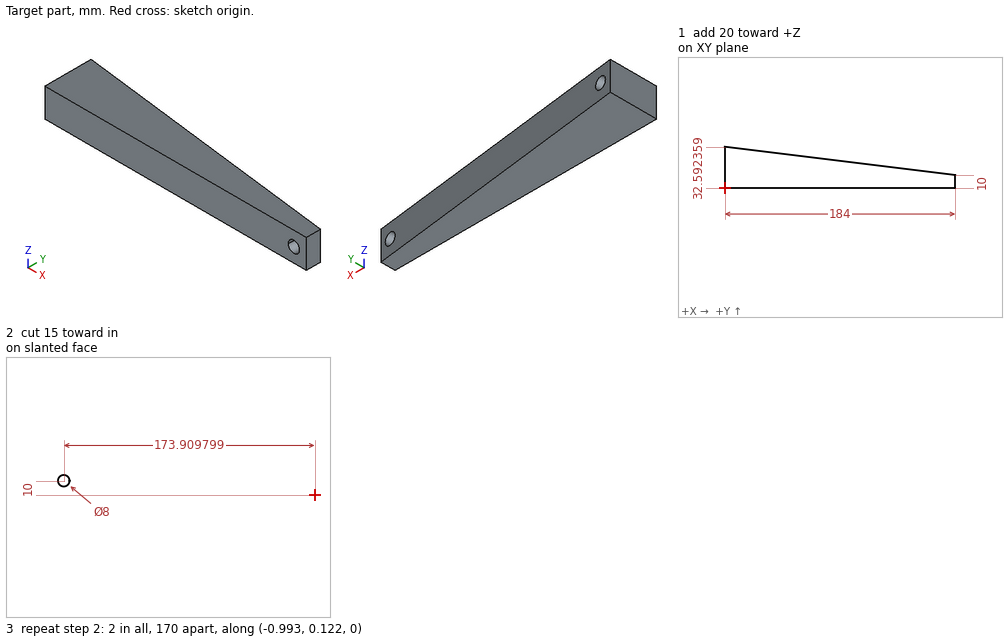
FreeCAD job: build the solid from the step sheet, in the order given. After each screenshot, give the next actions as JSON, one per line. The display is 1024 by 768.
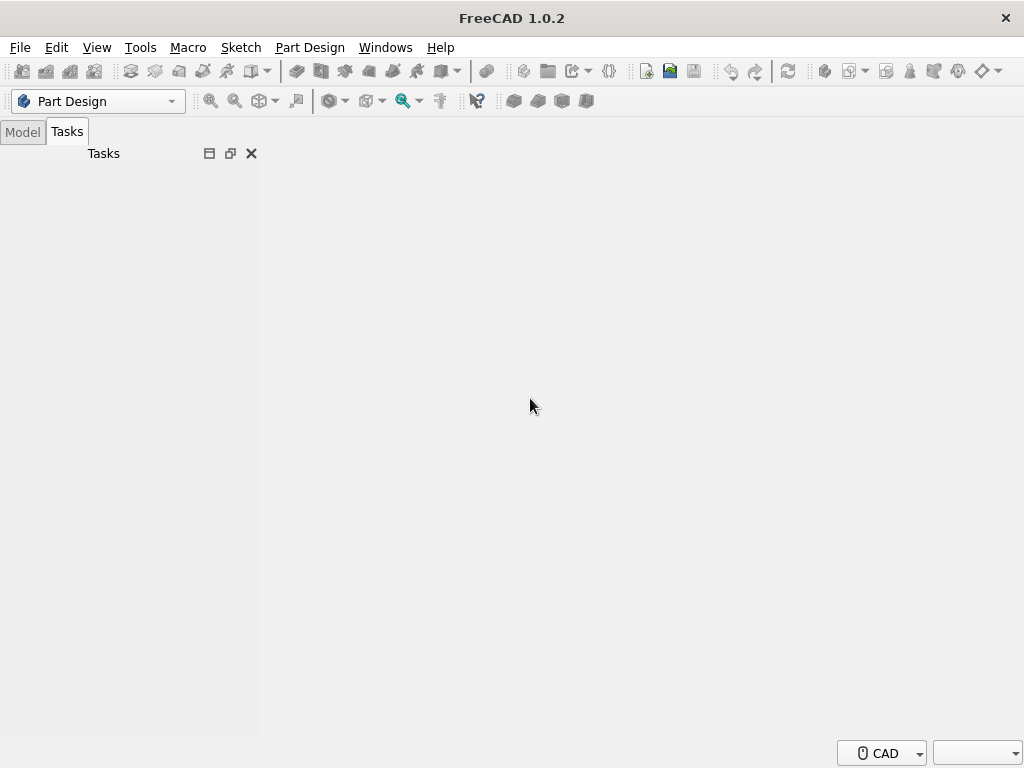
{"action": "left_click", "coordinate": [646, 72]}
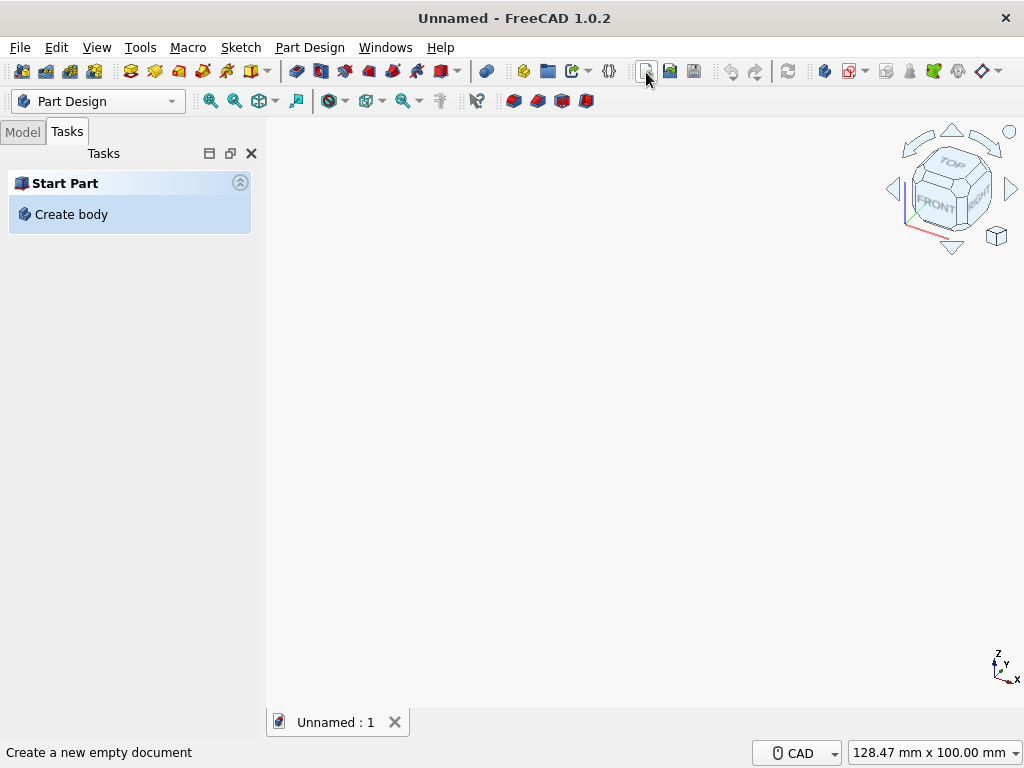
{"action": "left_click", "coordinate": [850, 72]}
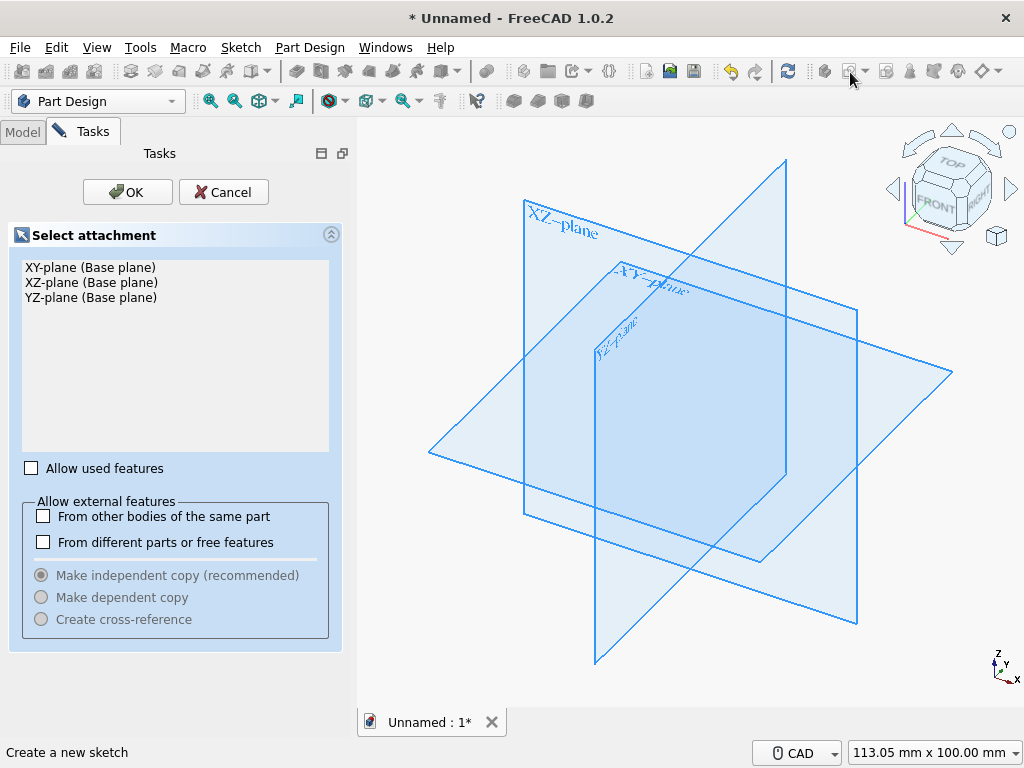
{"action": "left_click", "coordinate": [82, 268]}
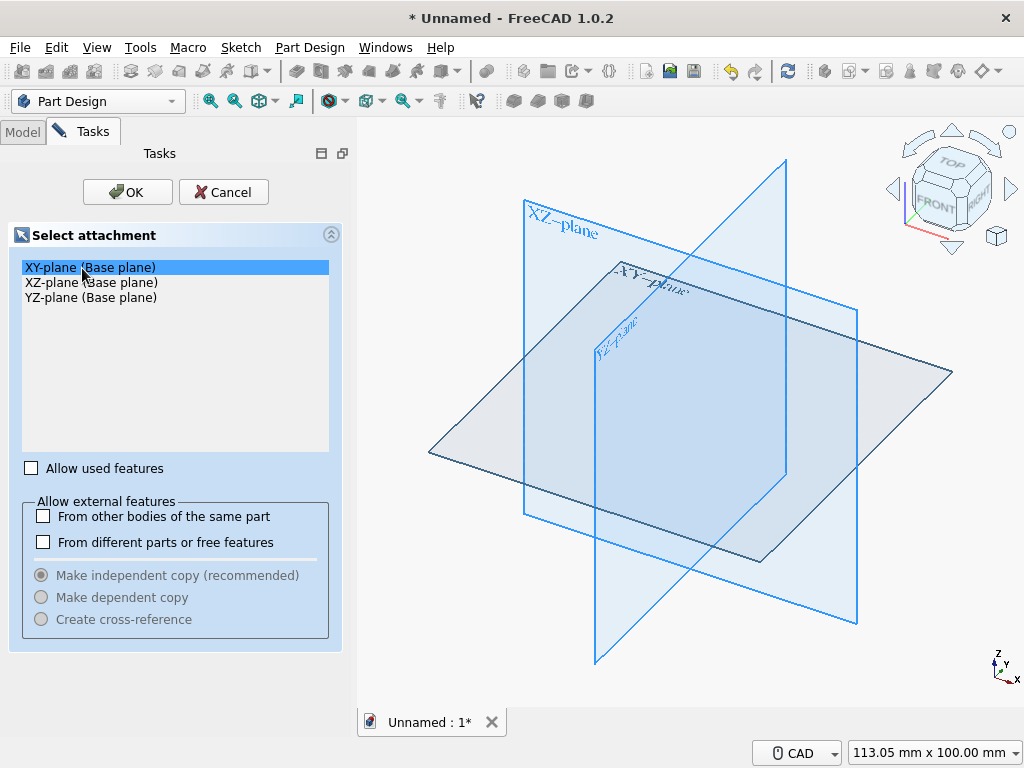
{"action": "left_click", "coordinate": [128, 192]}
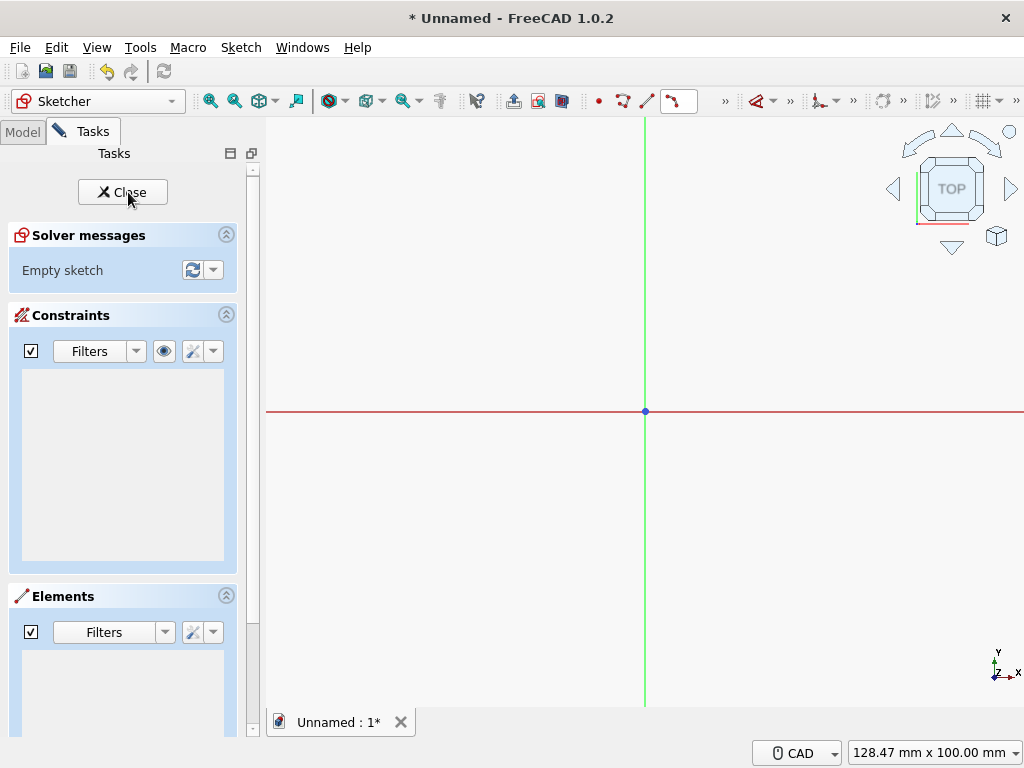
{"action": "scroll", "coordinate": [294, 468], "scroll_direction": "down", "scroll_amount": 5}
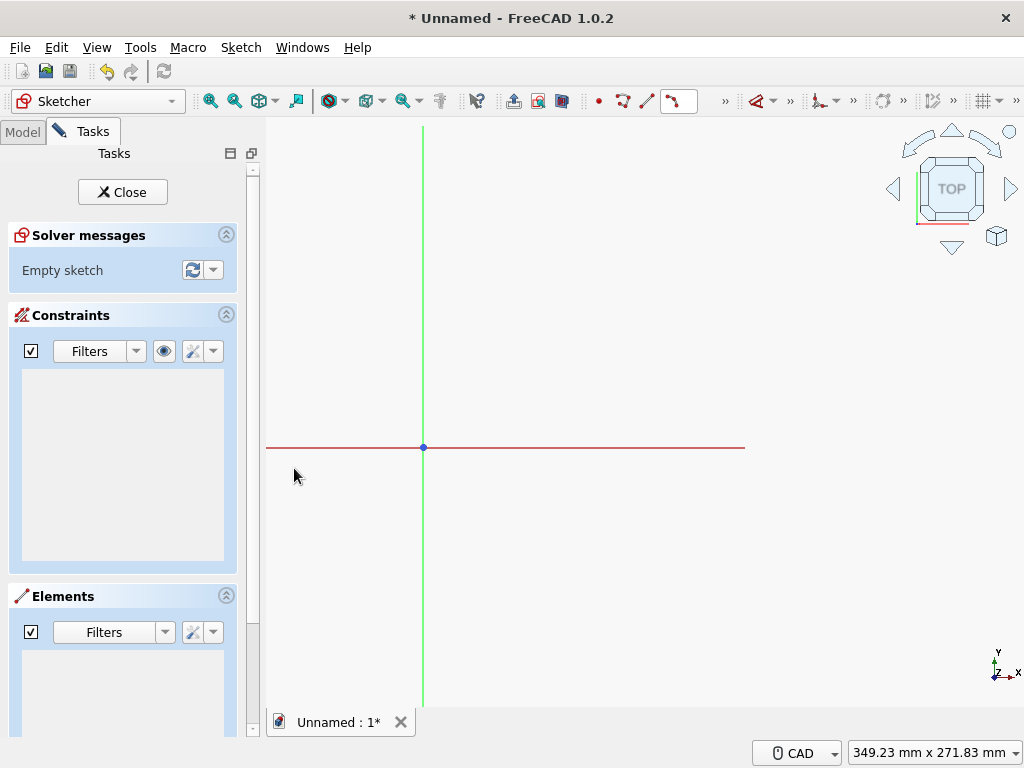
{"action": "left_click", "coordinate": [624, 102]}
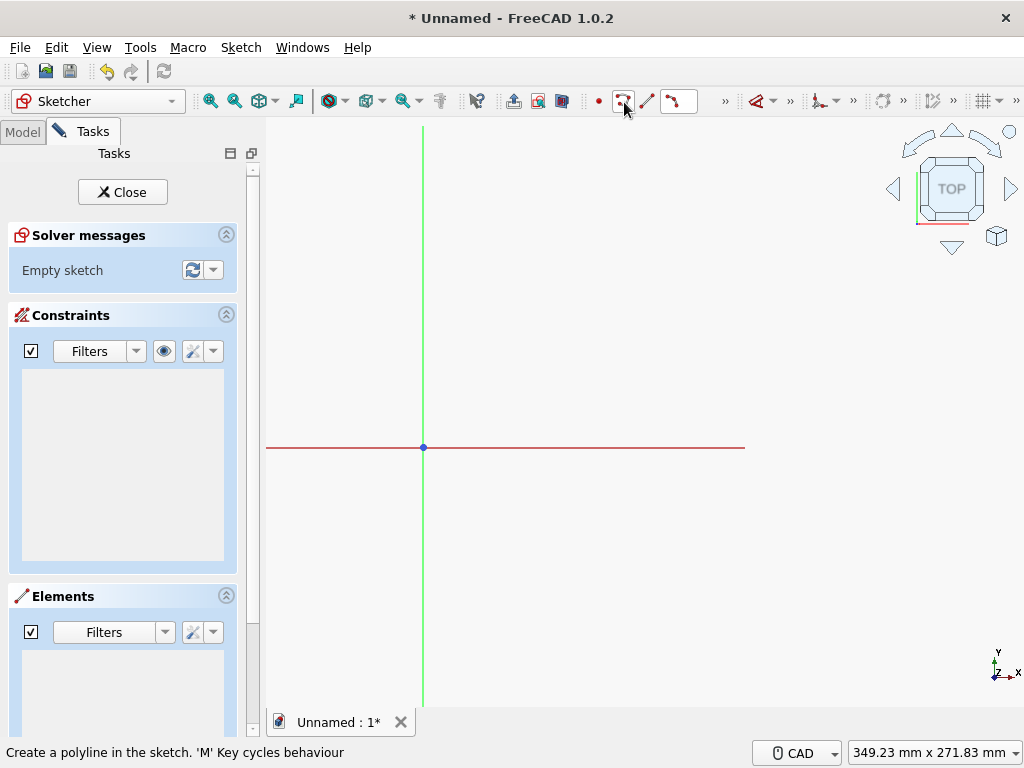
{"action": "left_click", "coordinate": [423, 448]}
{"action": "left_click", "coordinate": [823, 439]}
{"action": "left_click", "coordinate": [823, 426]}
{"action": "left_click", "coordinate": [432, 377]}
{"action": "left_click", "coordinate": [423, 448]}
{"action": "key", "text": "Escape"}
{"action": "key", "text": "Escape"}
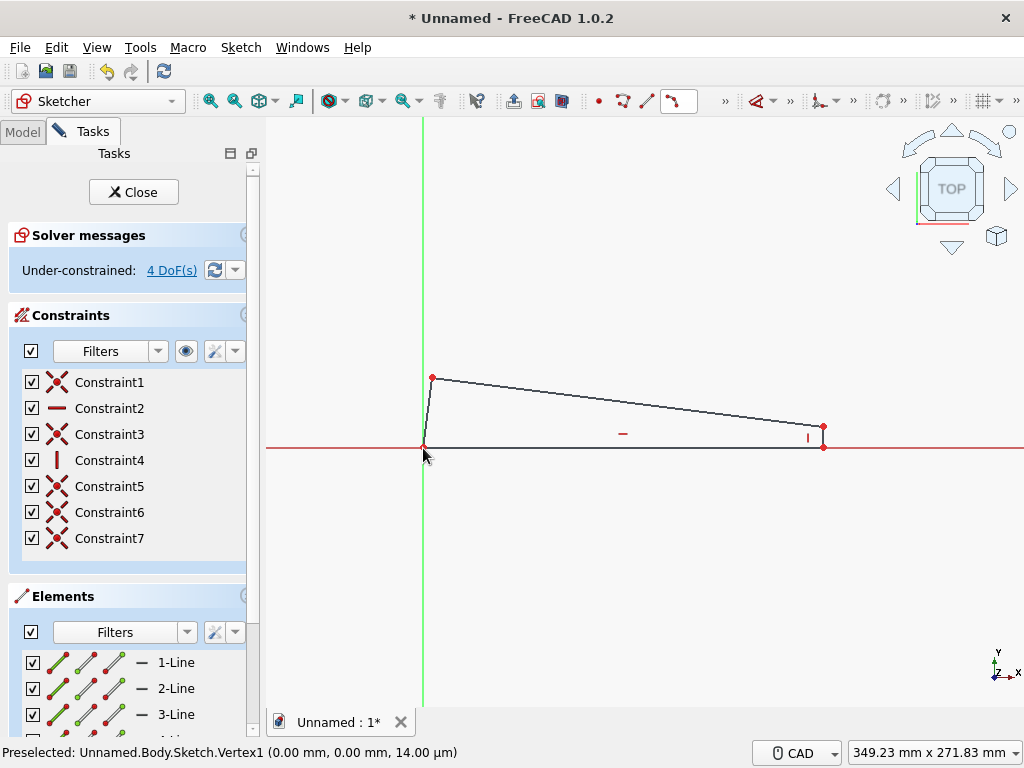
{"action": "left_click", "coordinate": [426, 427]}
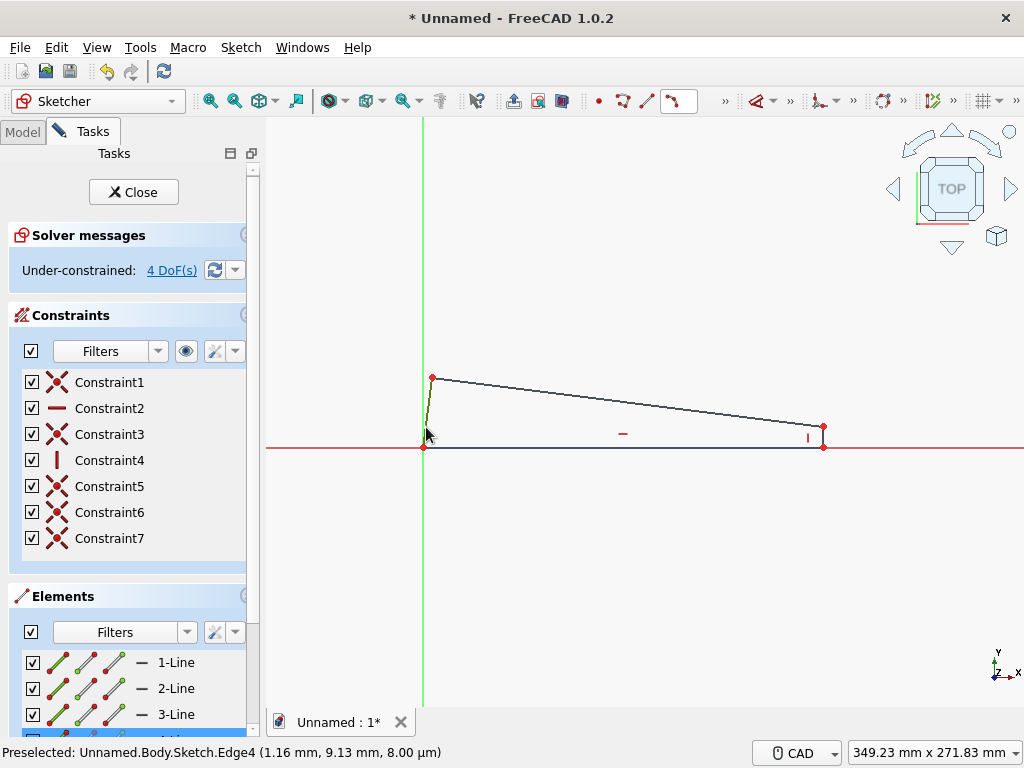
{"action": "key", "text": "v"}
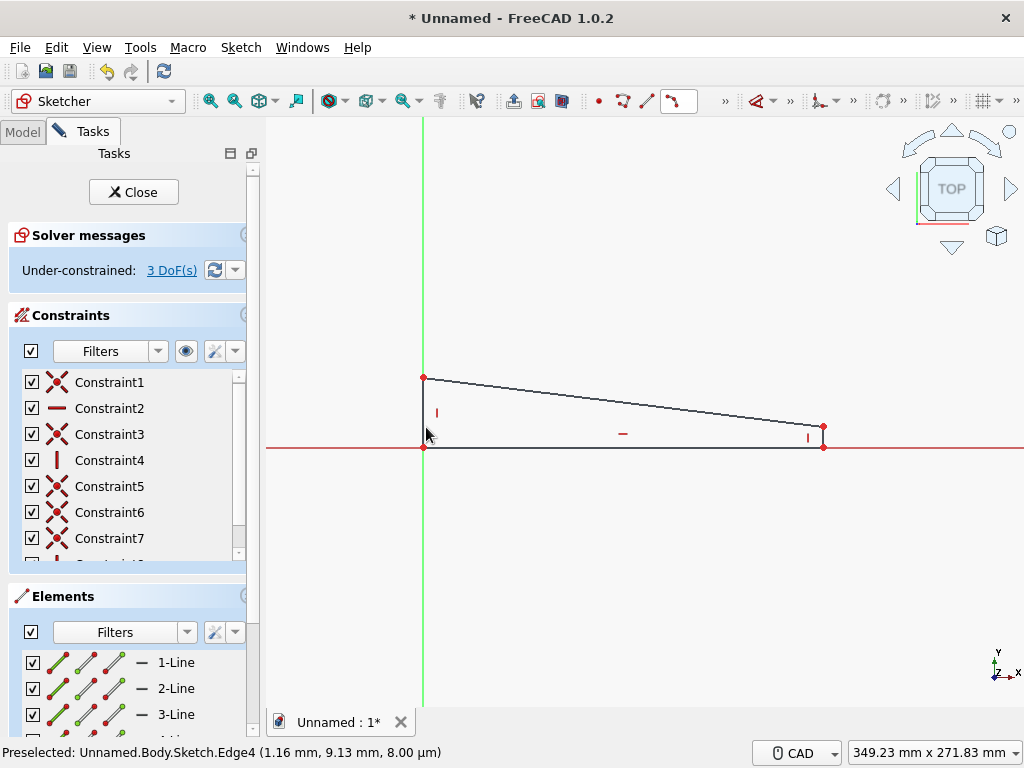
{"action": "scroll", "coordinate": [823, 437], "scroll_direction": "up", "scroll_amount": 4}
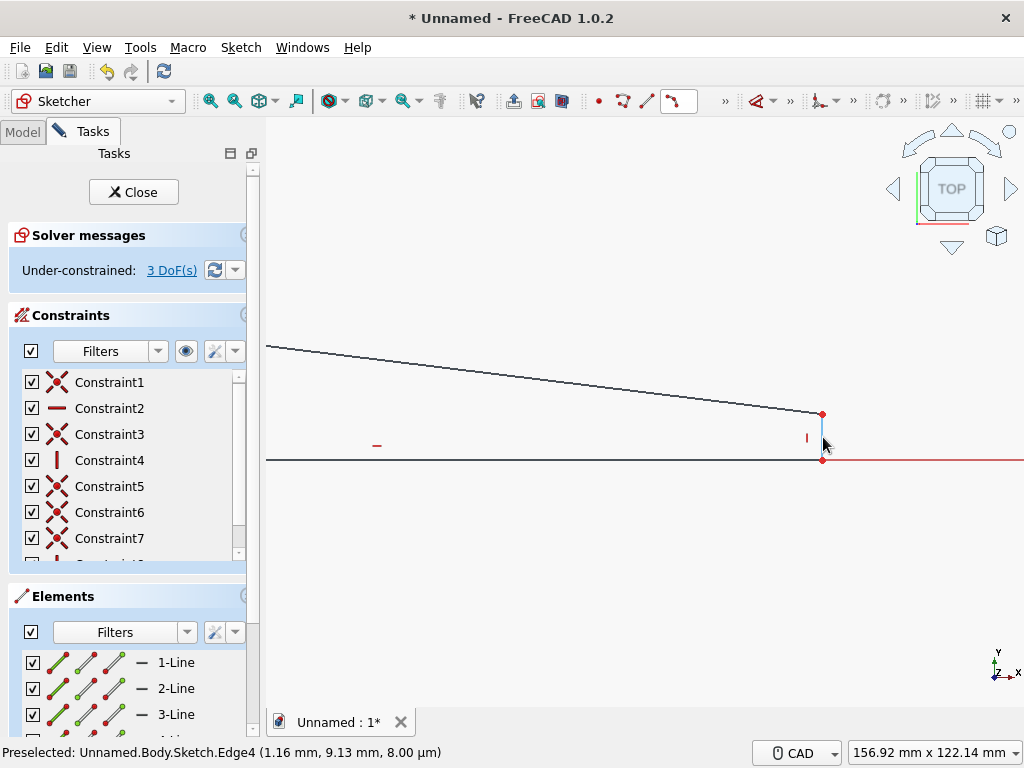
{"action": "left_click", "coordinate": [822, 437]}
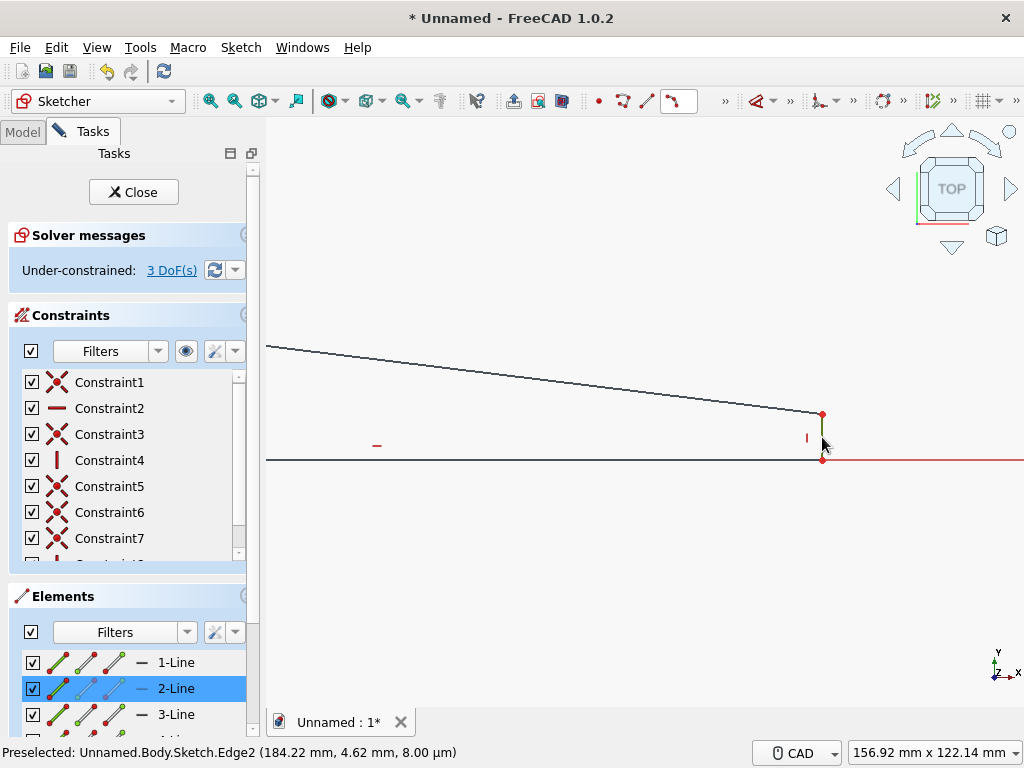
{"action": "key", "text": "i"}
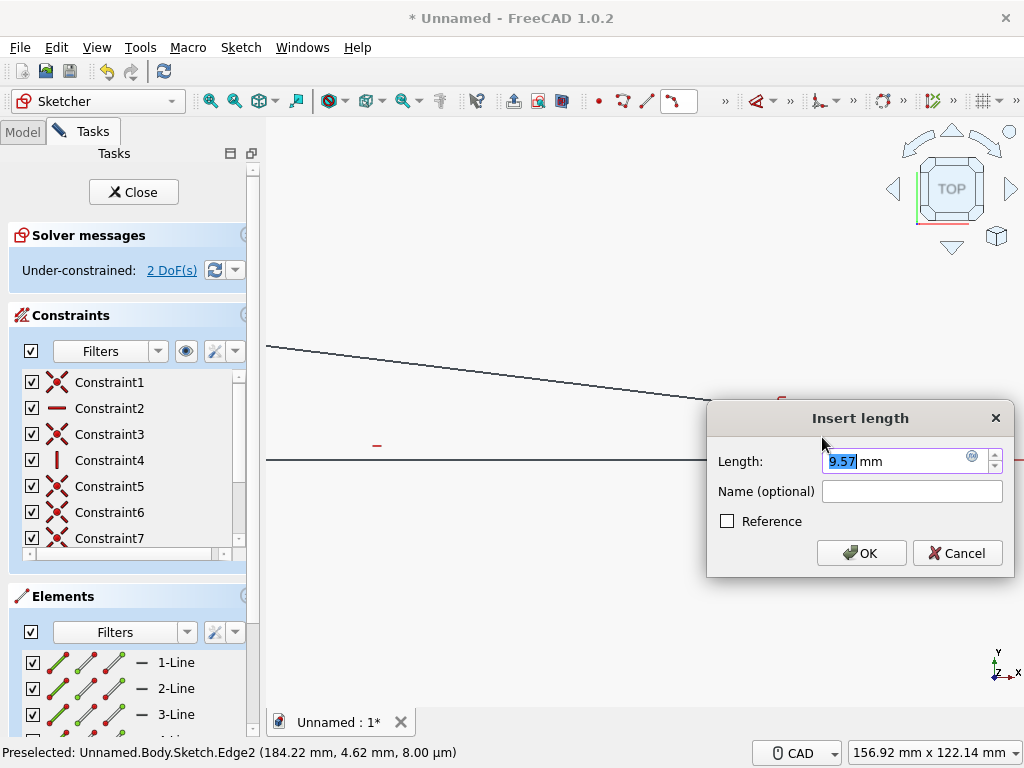
{"action": "type", "text": "10"}
{"action": "key", "text": "Return"}